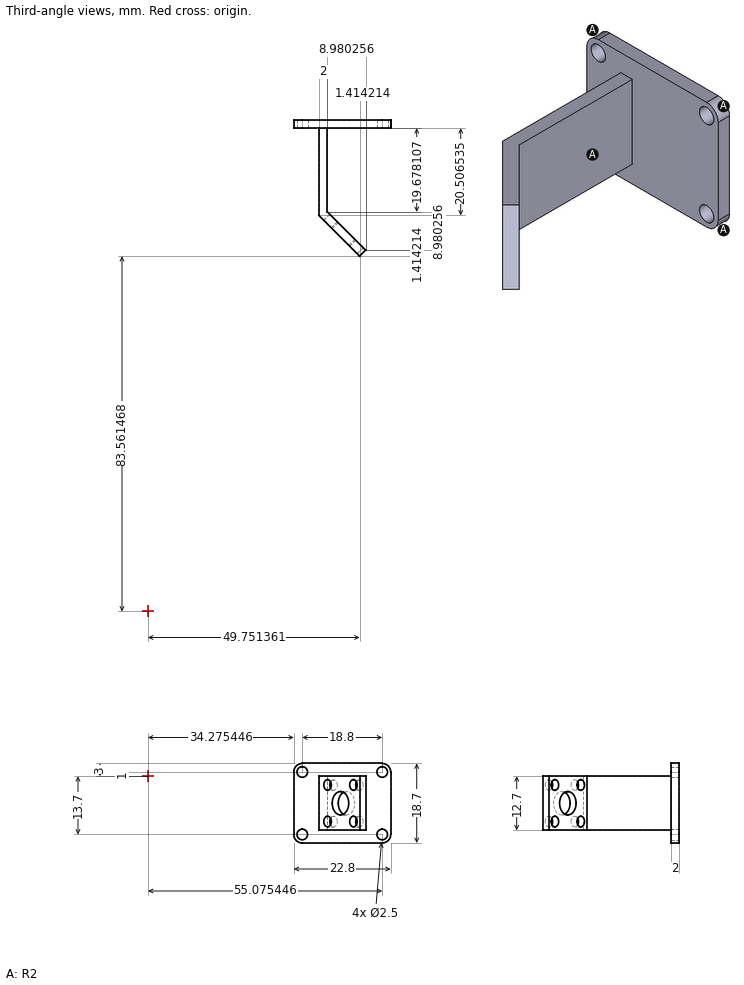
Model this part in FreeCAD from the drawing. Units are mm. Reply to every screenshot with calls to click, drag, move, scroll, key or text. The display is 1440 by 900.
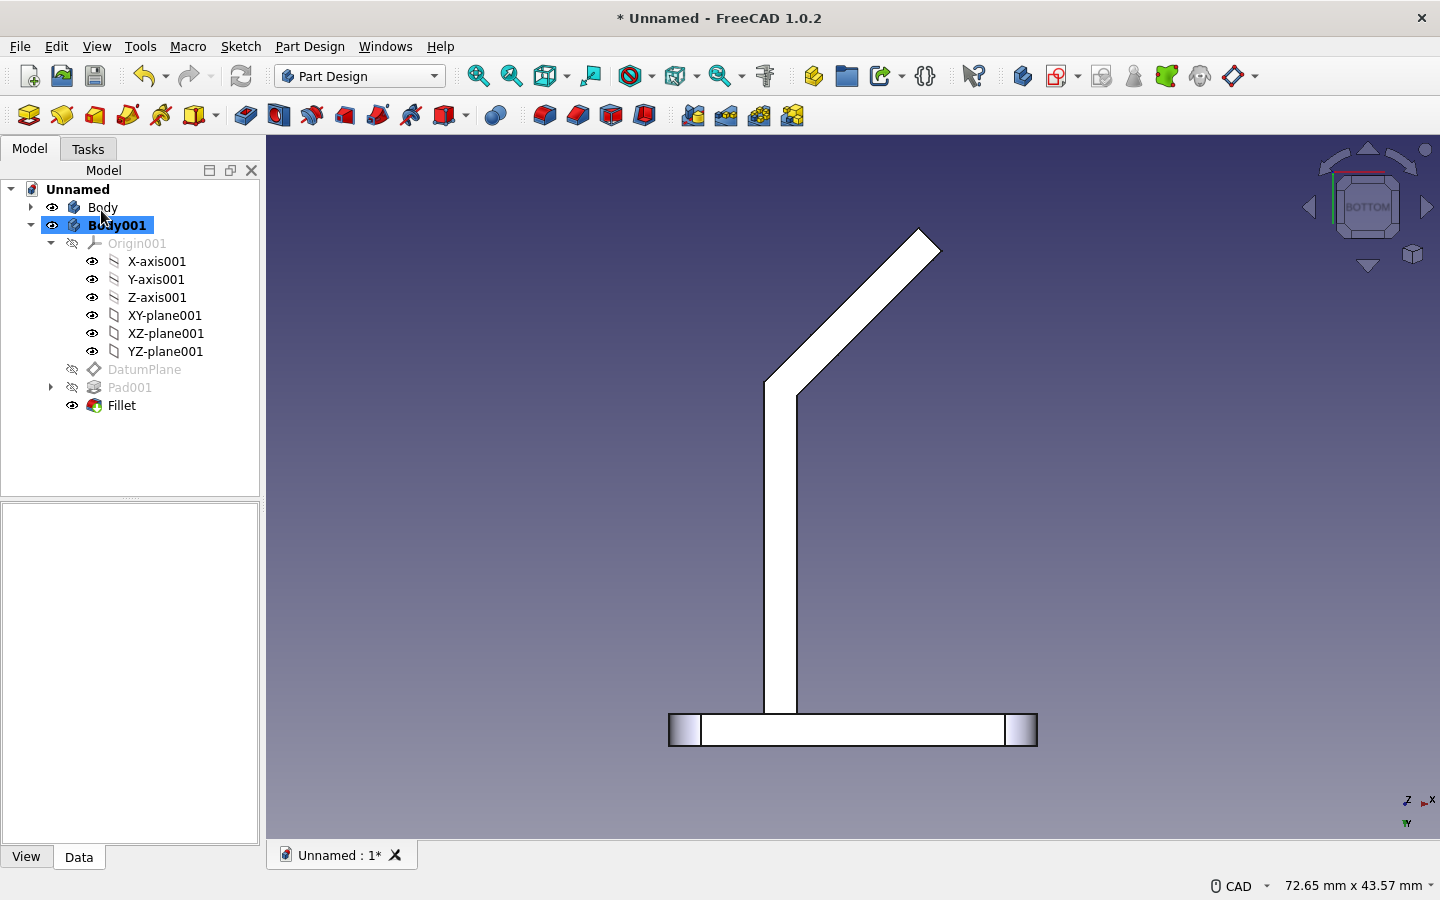
click(479, 76)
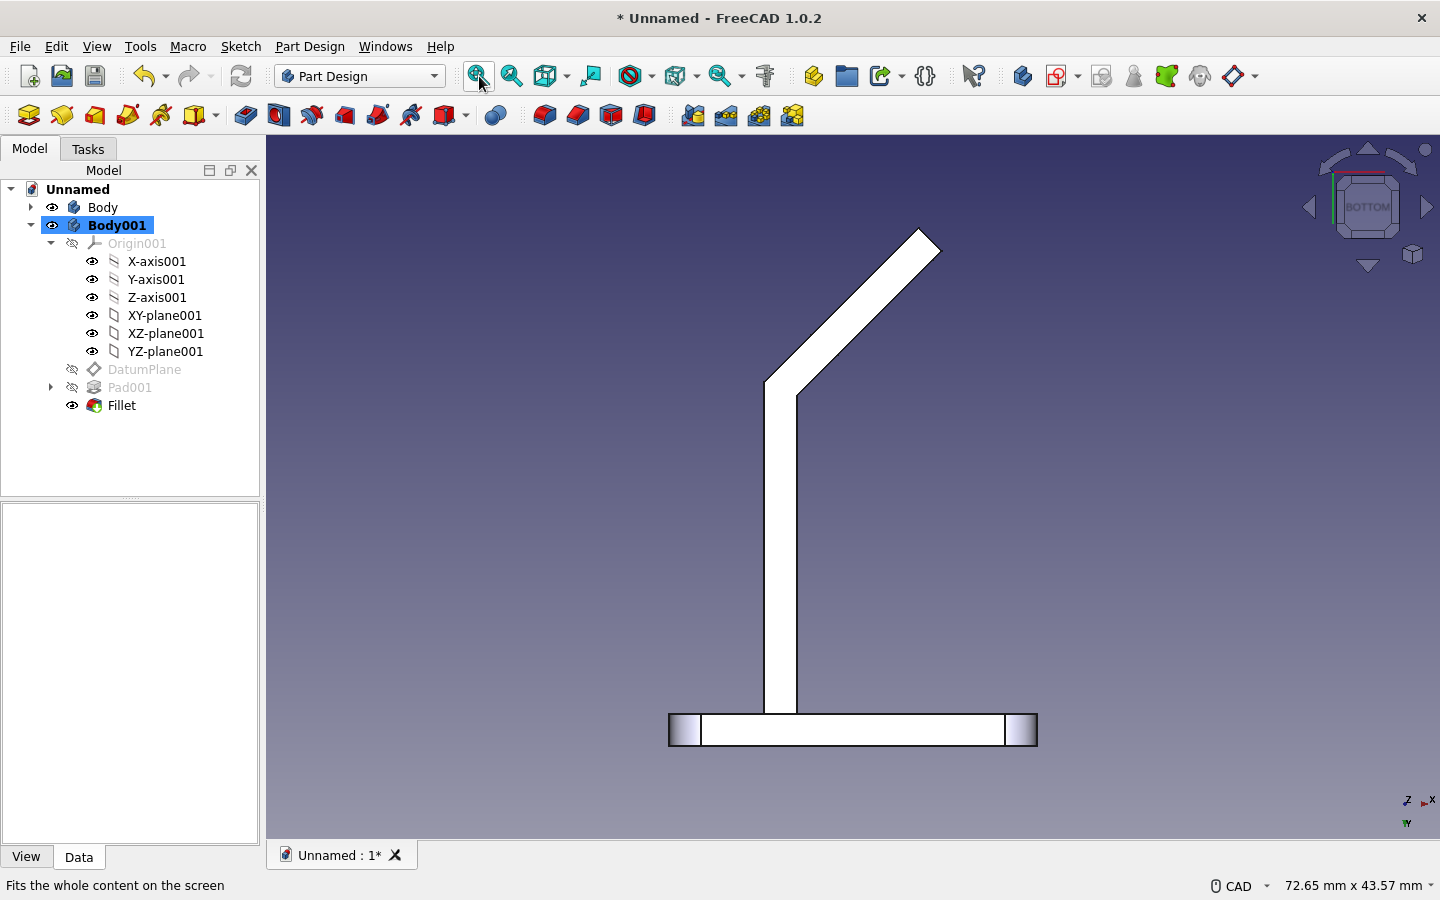
key(4)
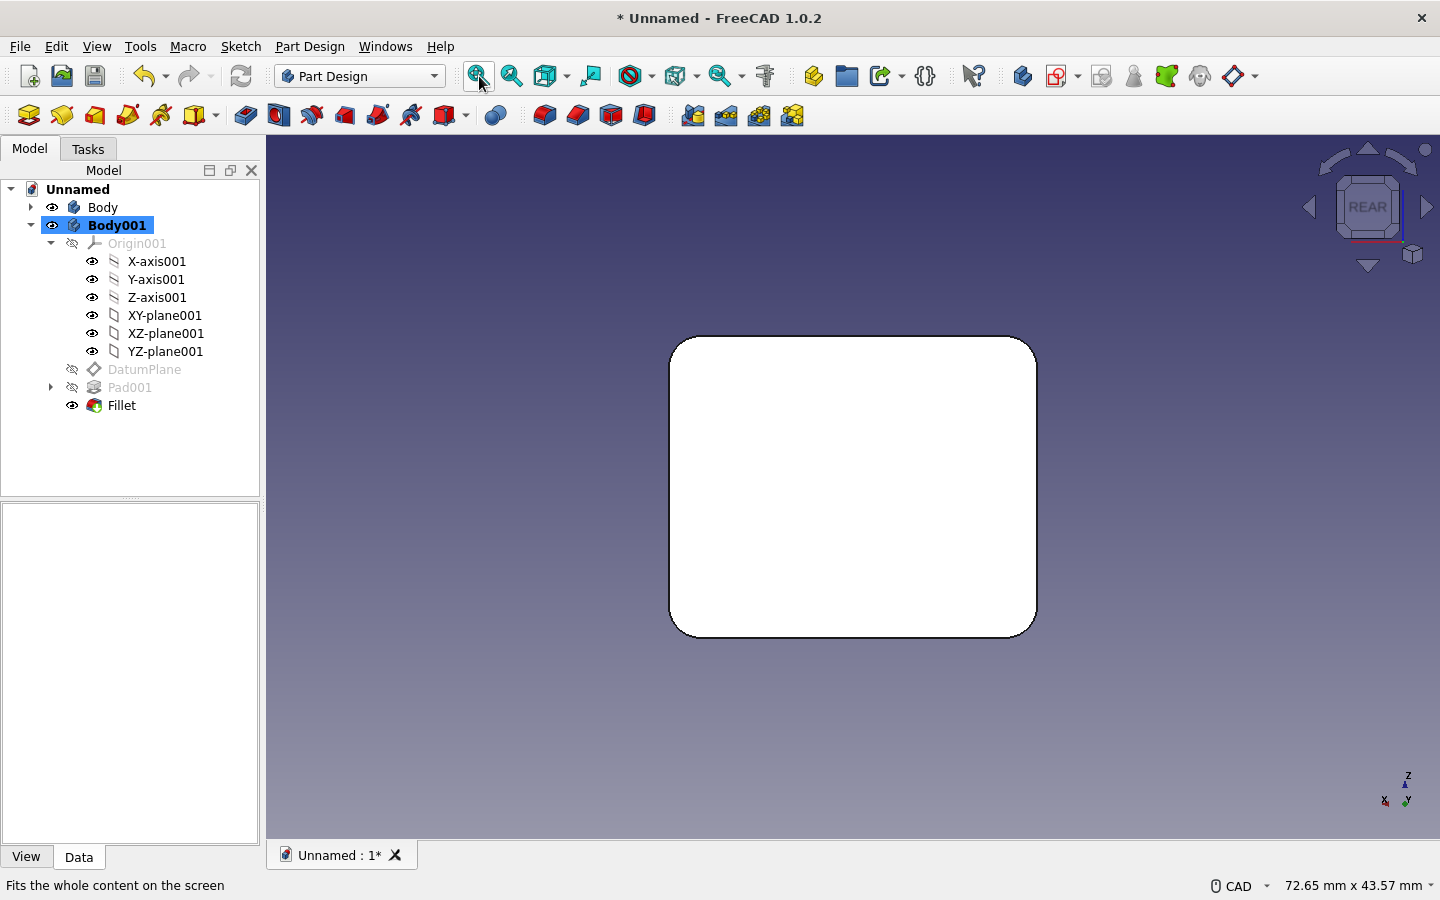
click(479, 76)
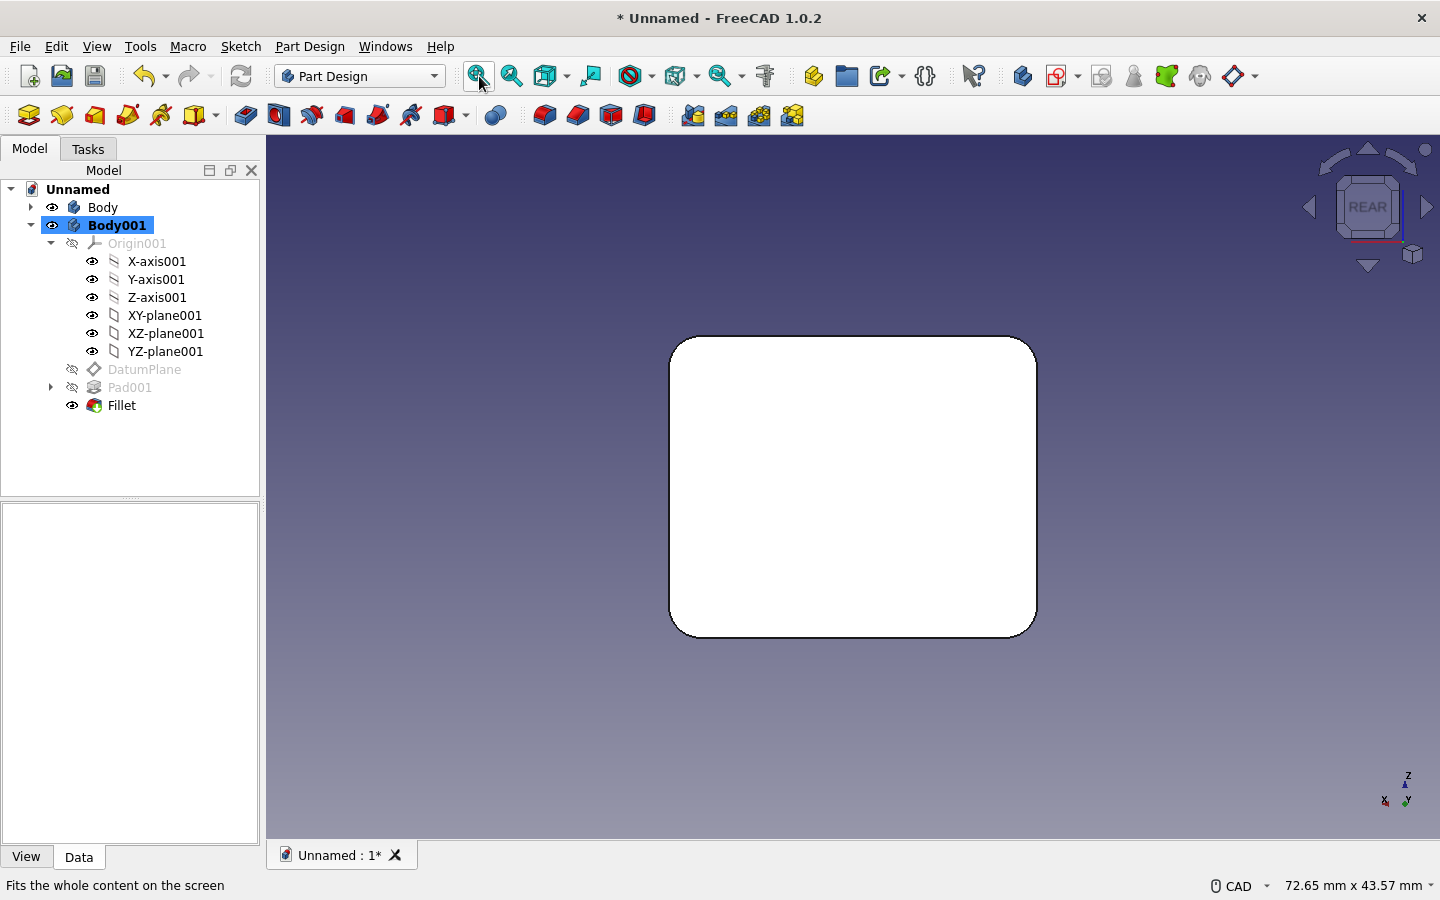
click(853, 486)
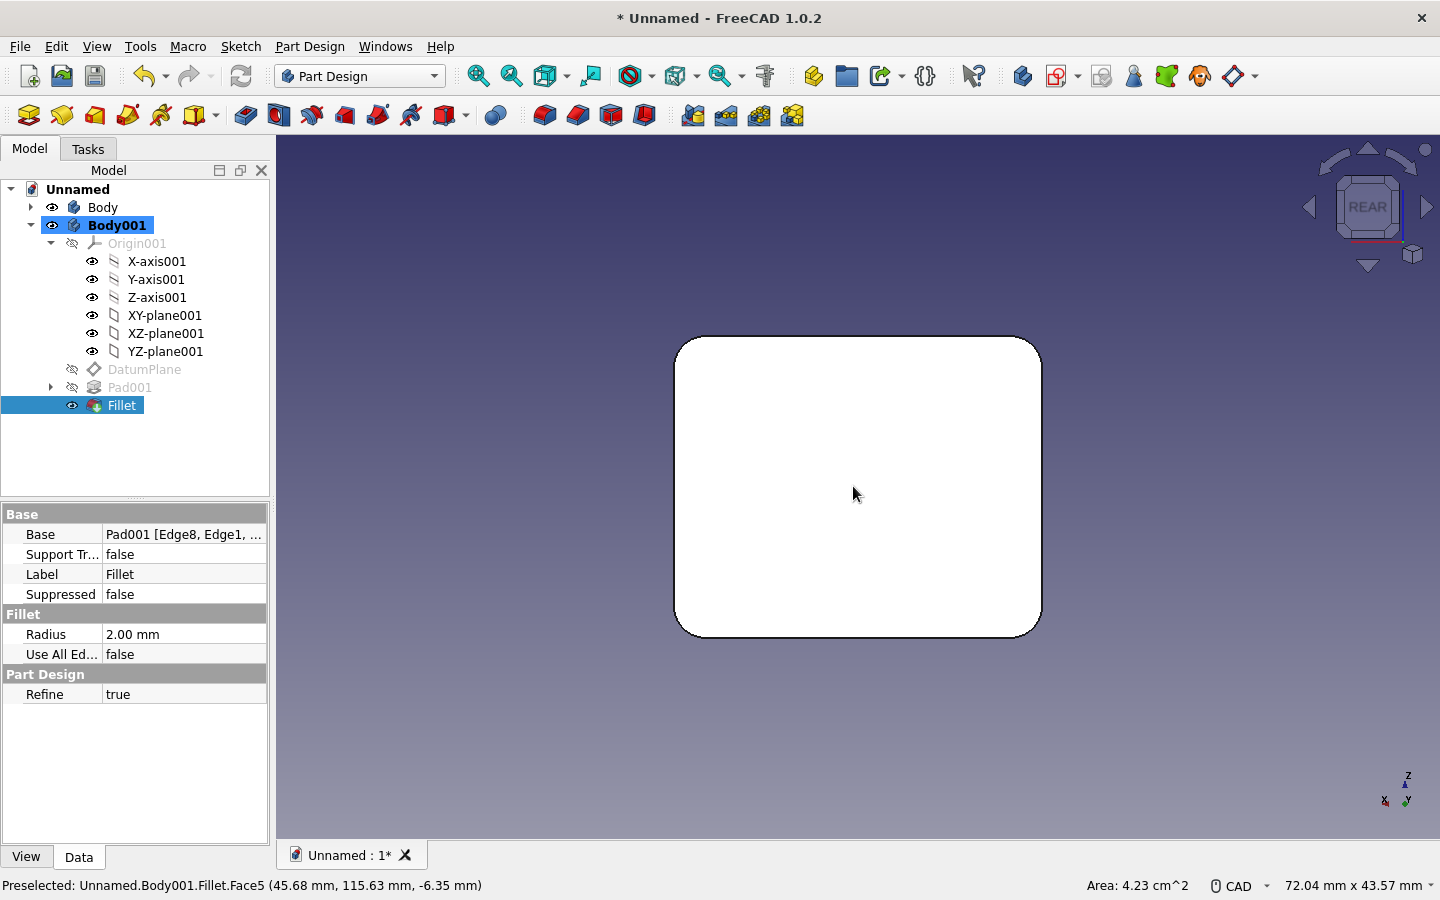
click(1056, 76)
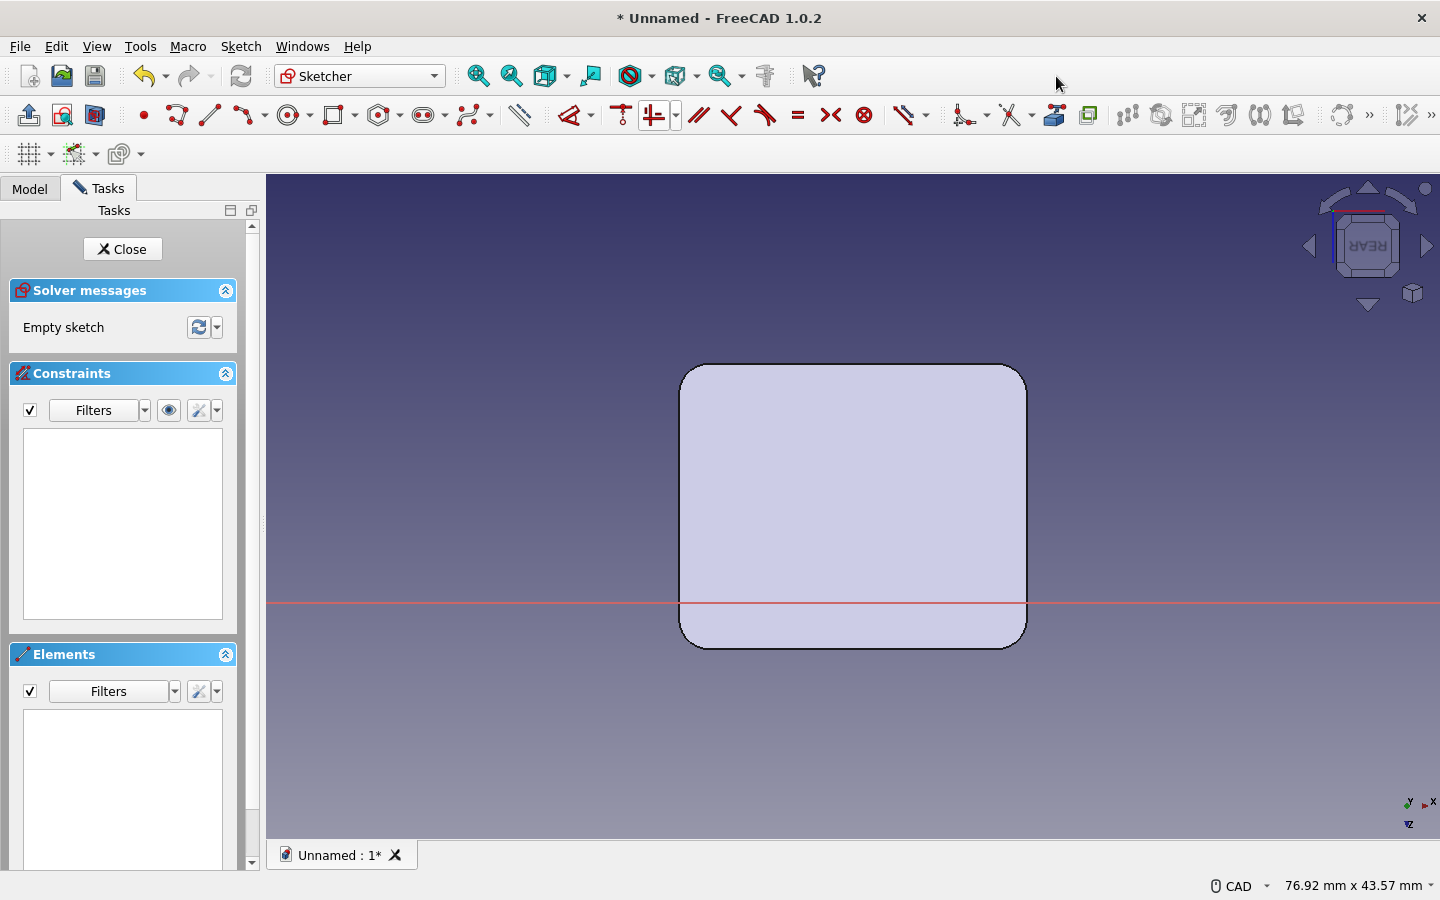
scroll(992, 507, up, 2)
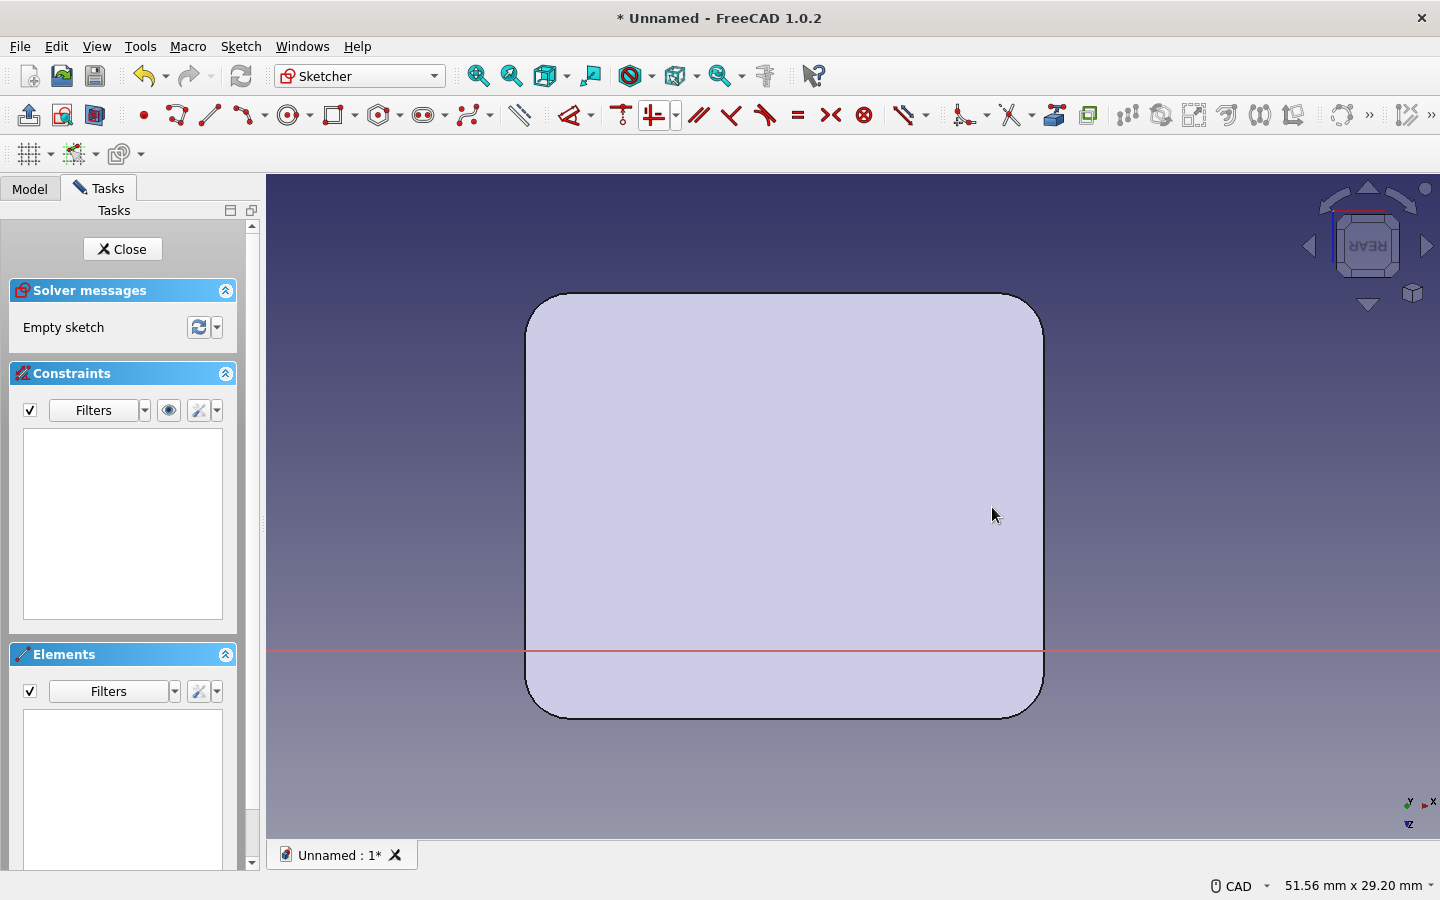
click(288, 116)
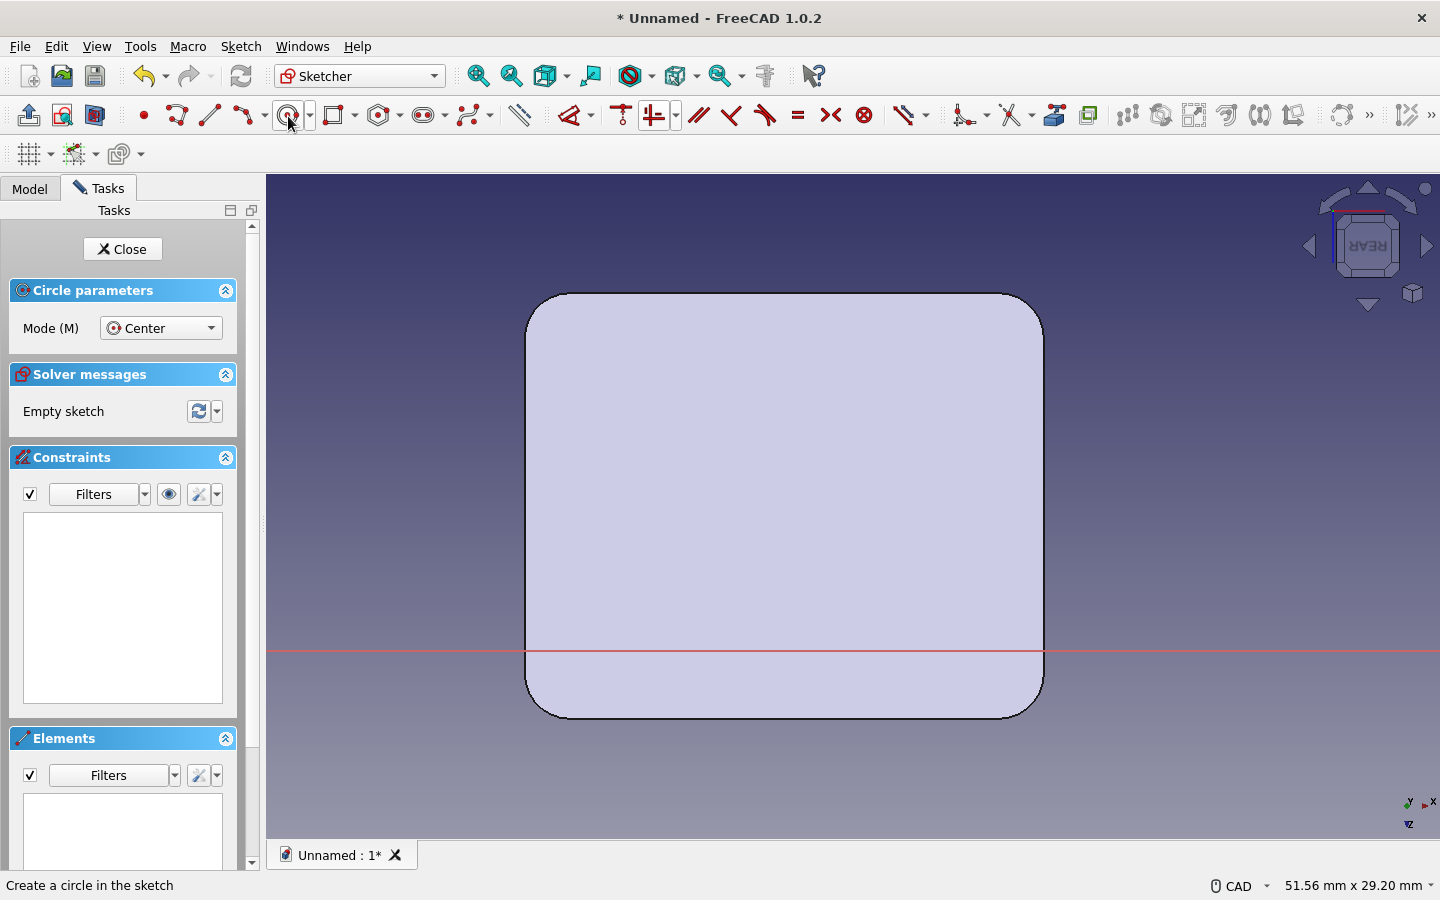
click(998, 339)
move(1019, 319)